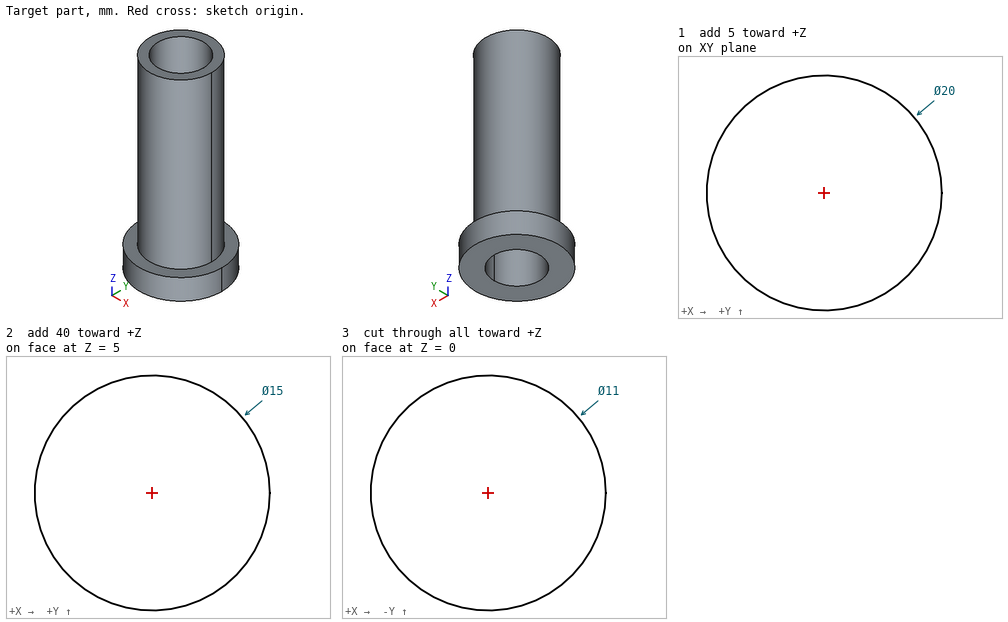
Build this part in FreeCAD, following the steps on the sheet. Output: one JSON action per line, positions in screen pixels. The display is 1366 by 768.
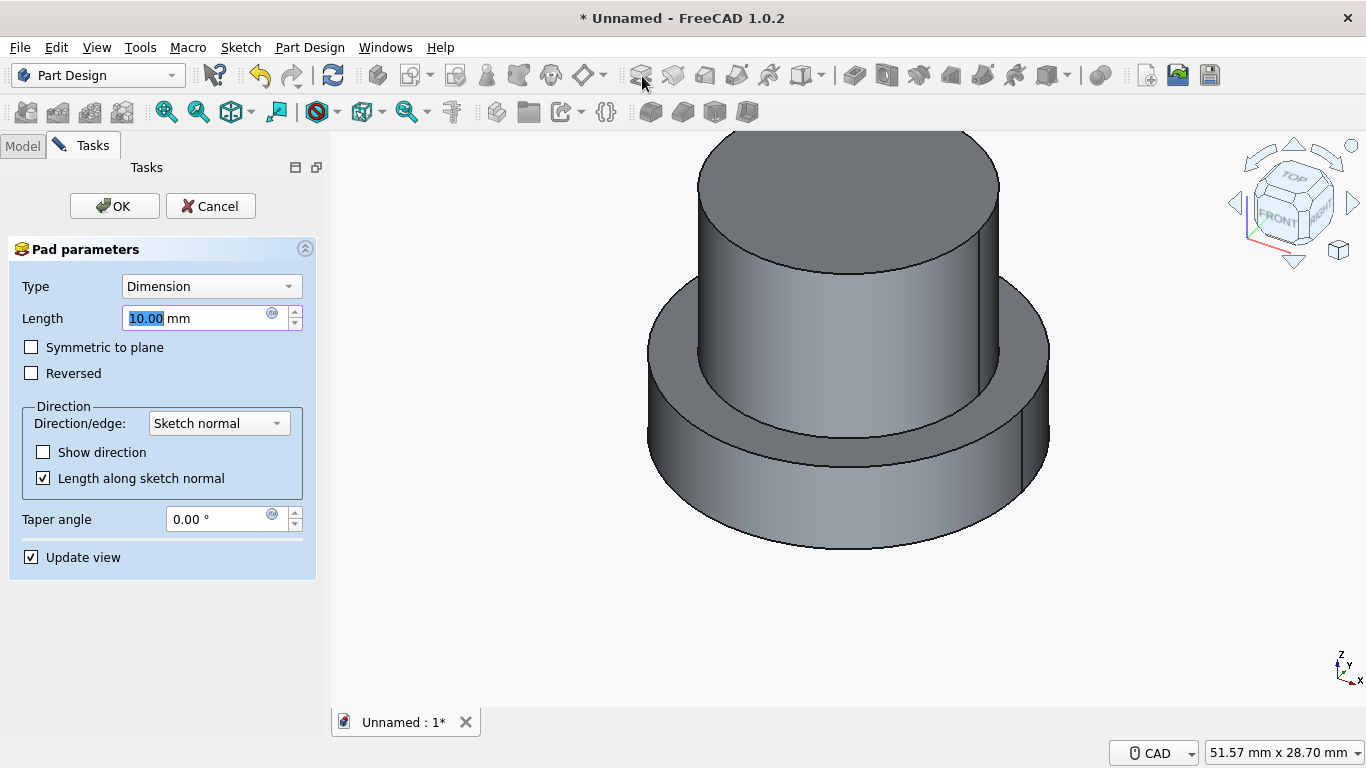
{"action": "type", "text": "40"}
{"action": "key", "text": "Tab"}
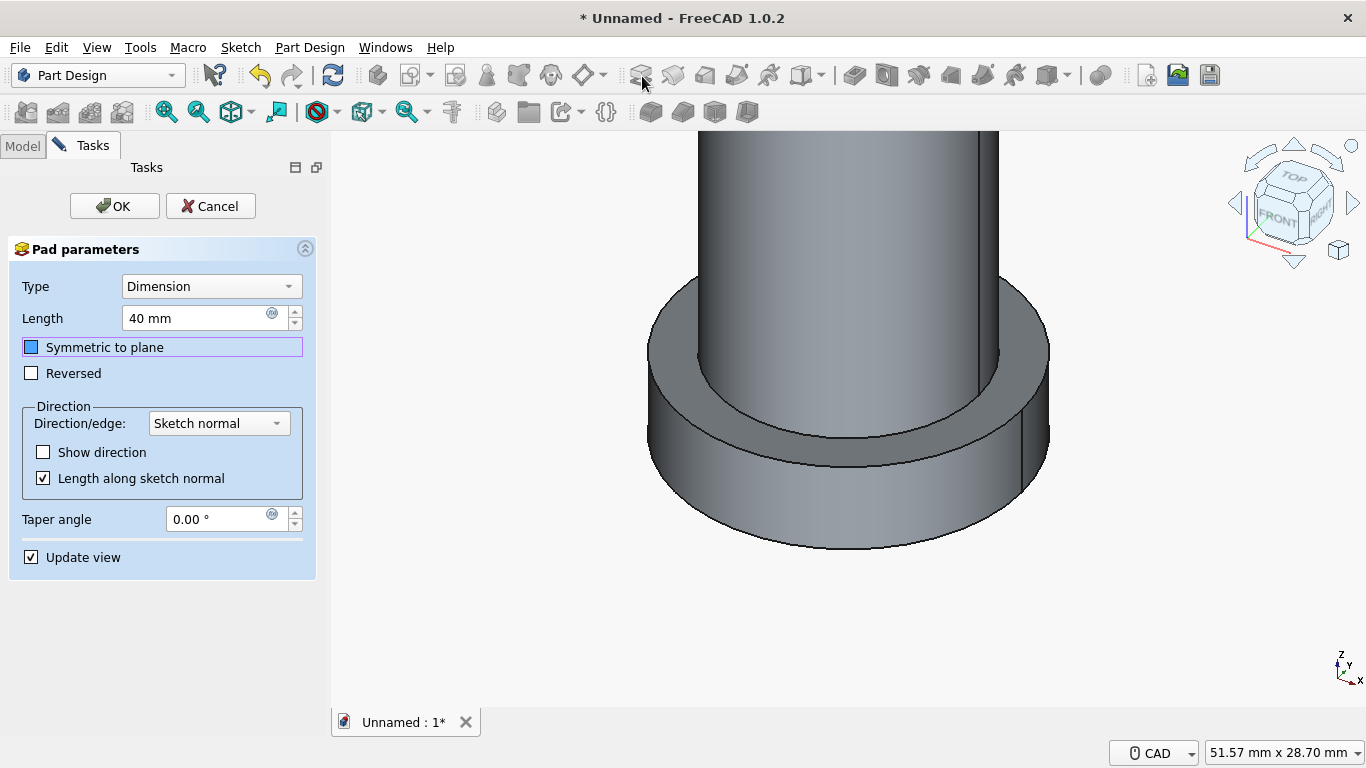
{"action": "left_click", "coordinate": [115, 206]}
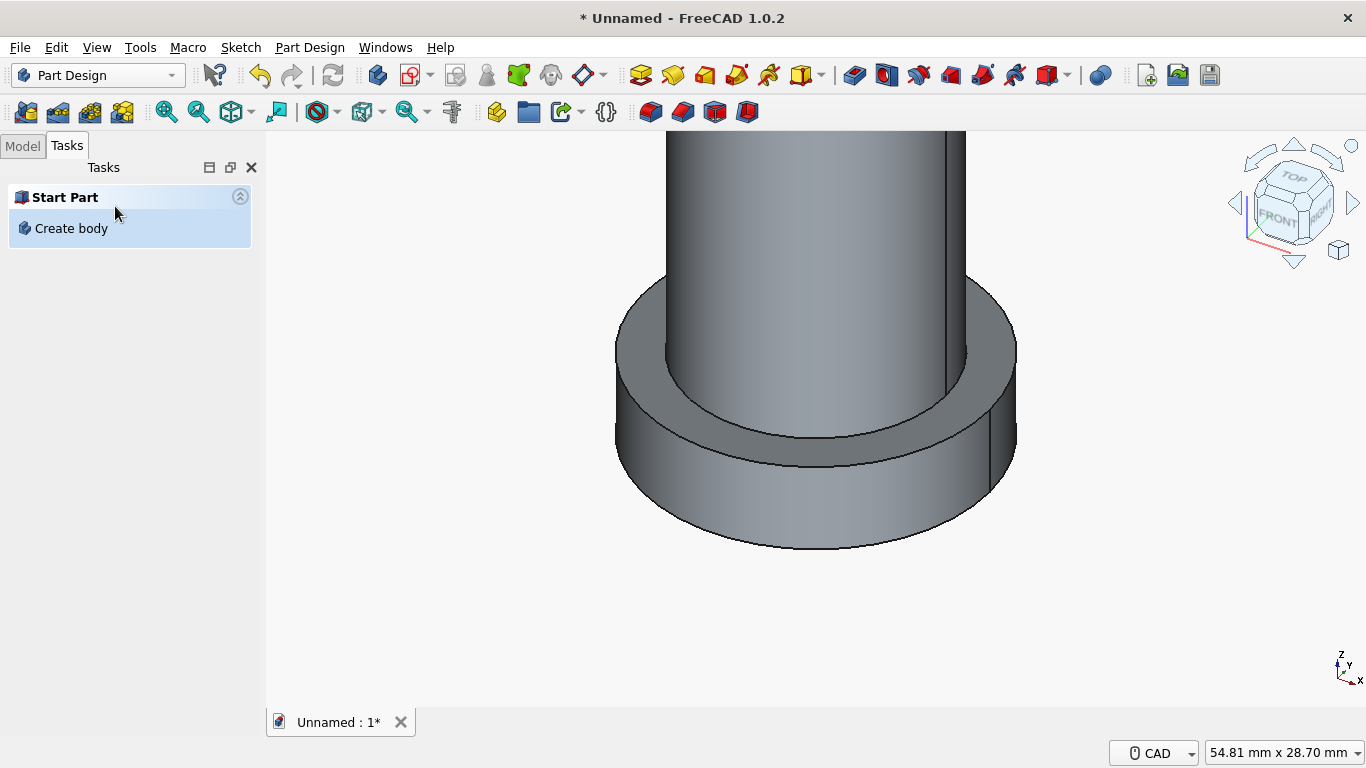
{"action": "left_click", "coordinate": [168, 112]}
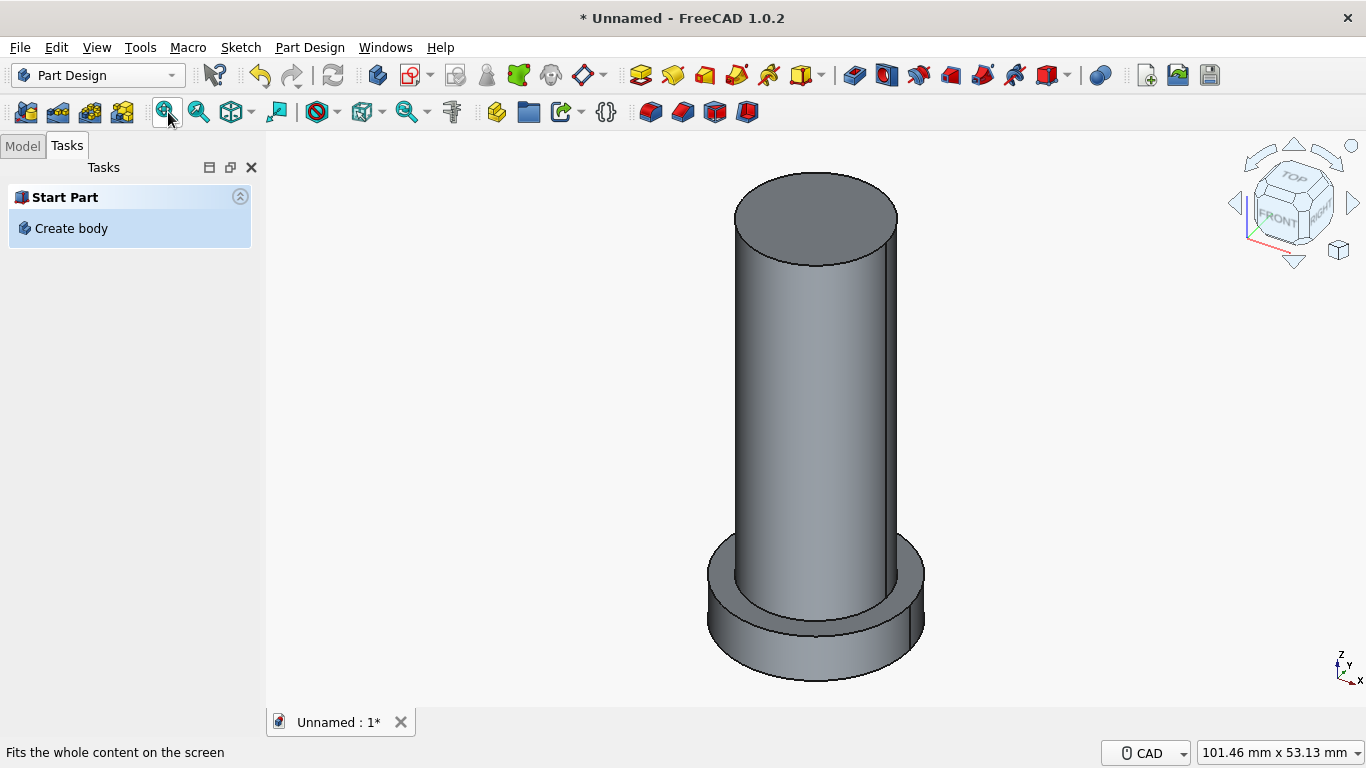
{"action": "key", "text": "5"}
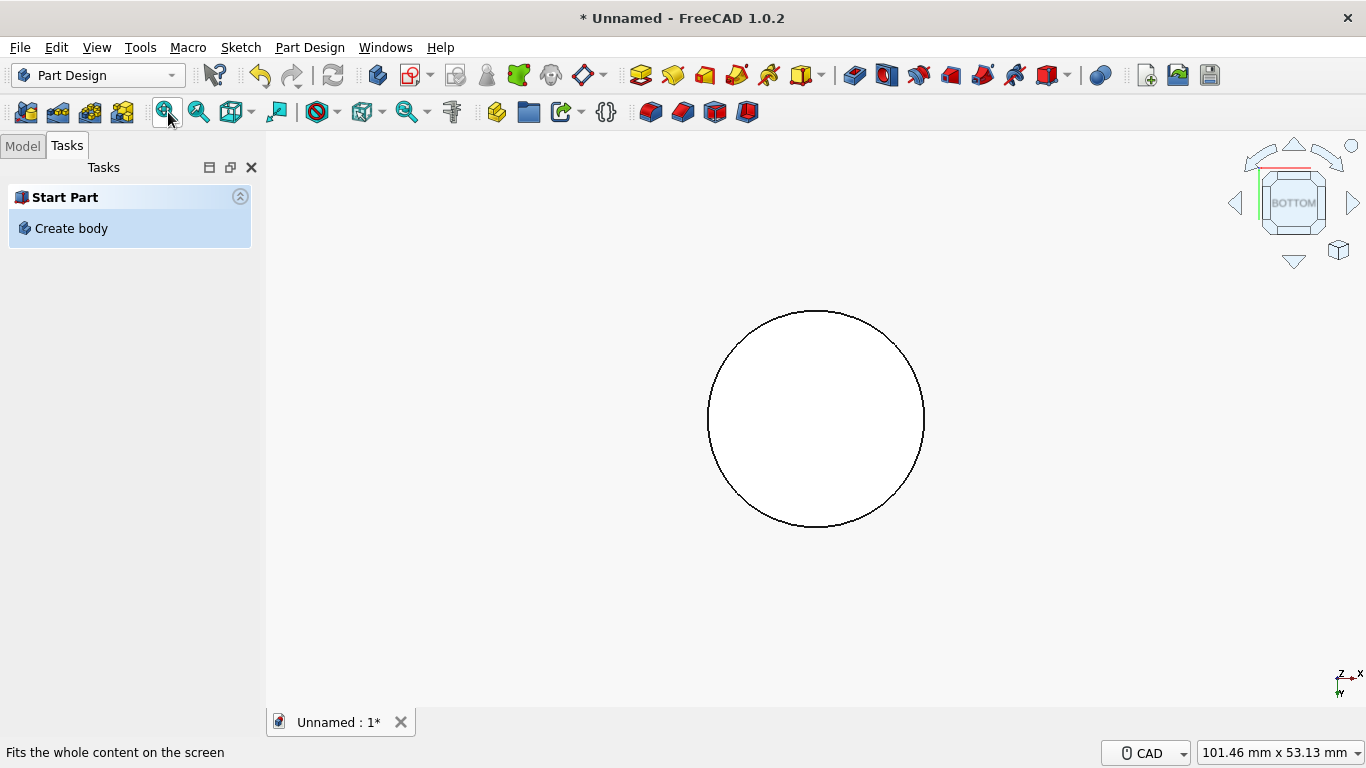
{"action": "key", "text": "v f"}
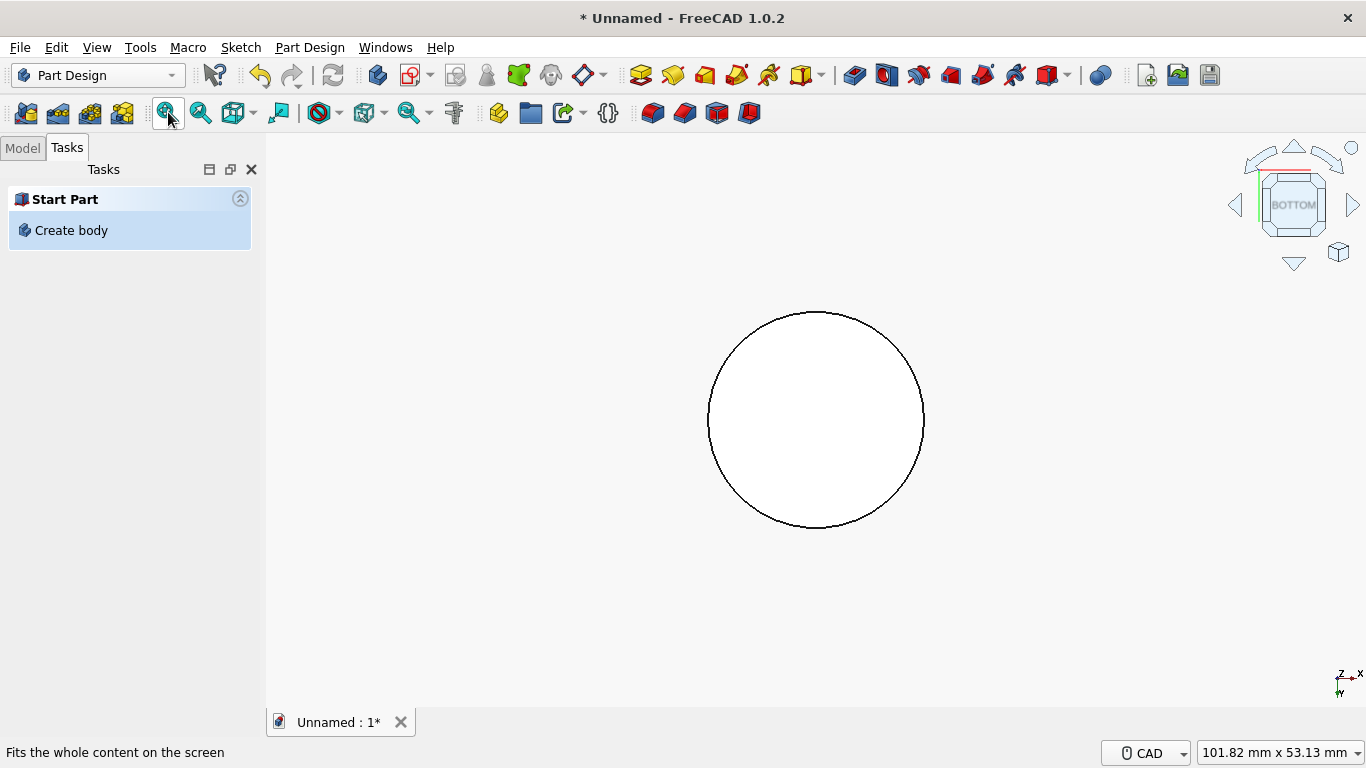
{"action": "left_click", "coordinate": [816, 419]}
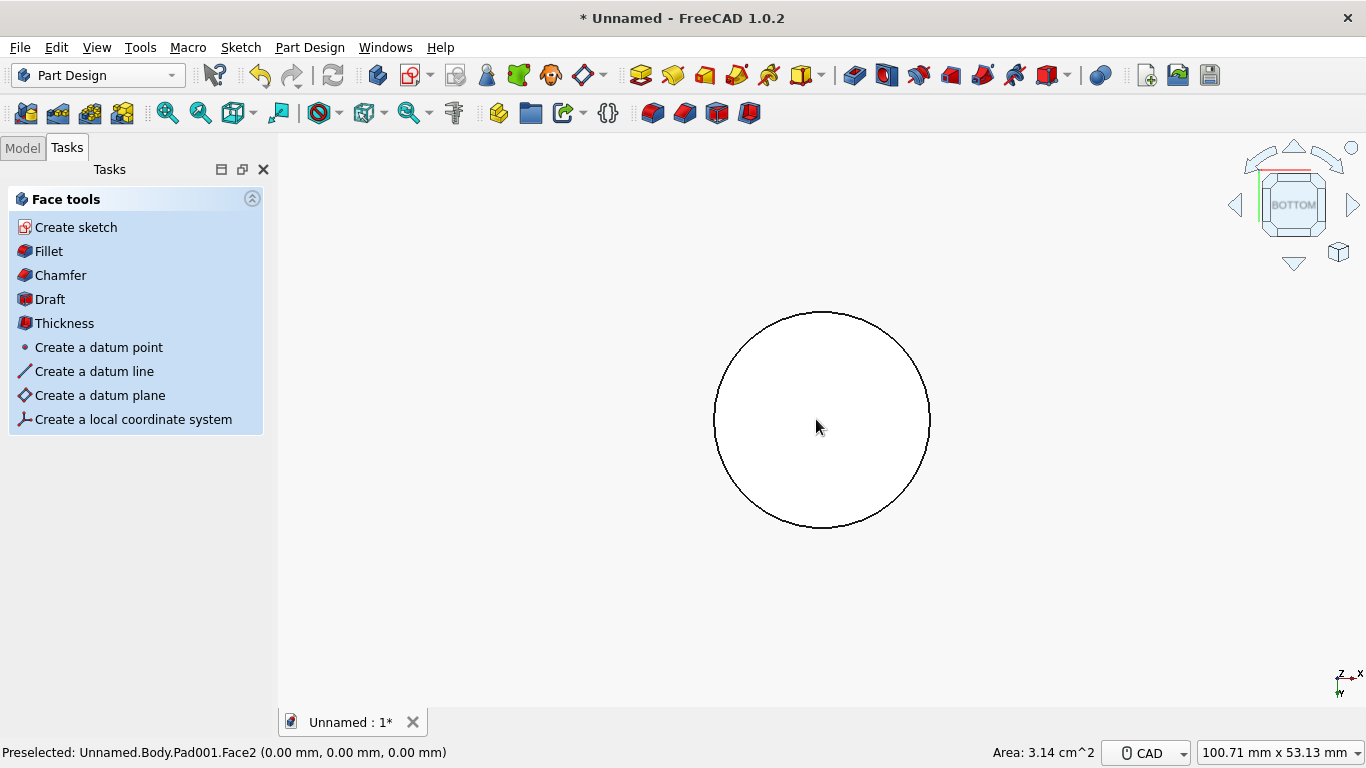
{"action": "left_click", "coordinate": [410, 76]}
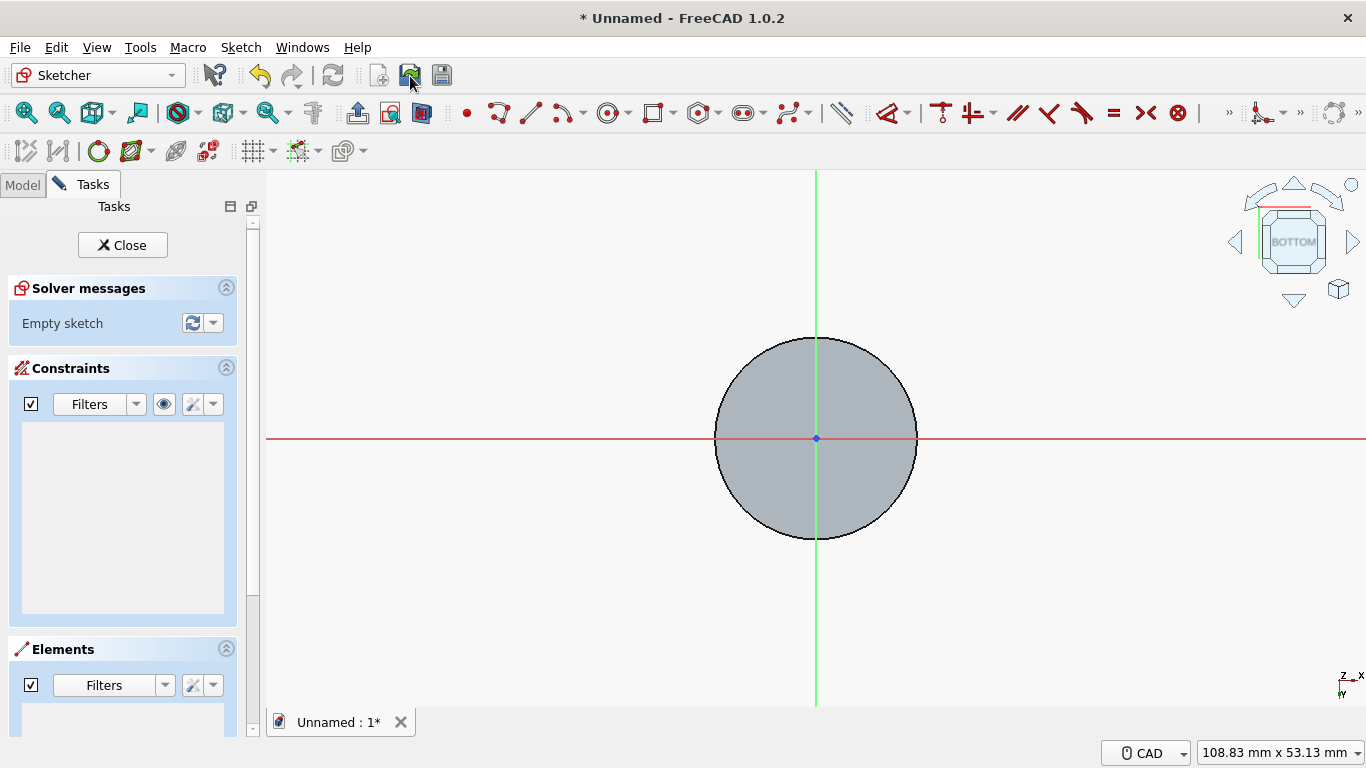
{"action": "scroll", "coordinate": [846, 438], "scroll_direction": "up", "scroll_amount": 6}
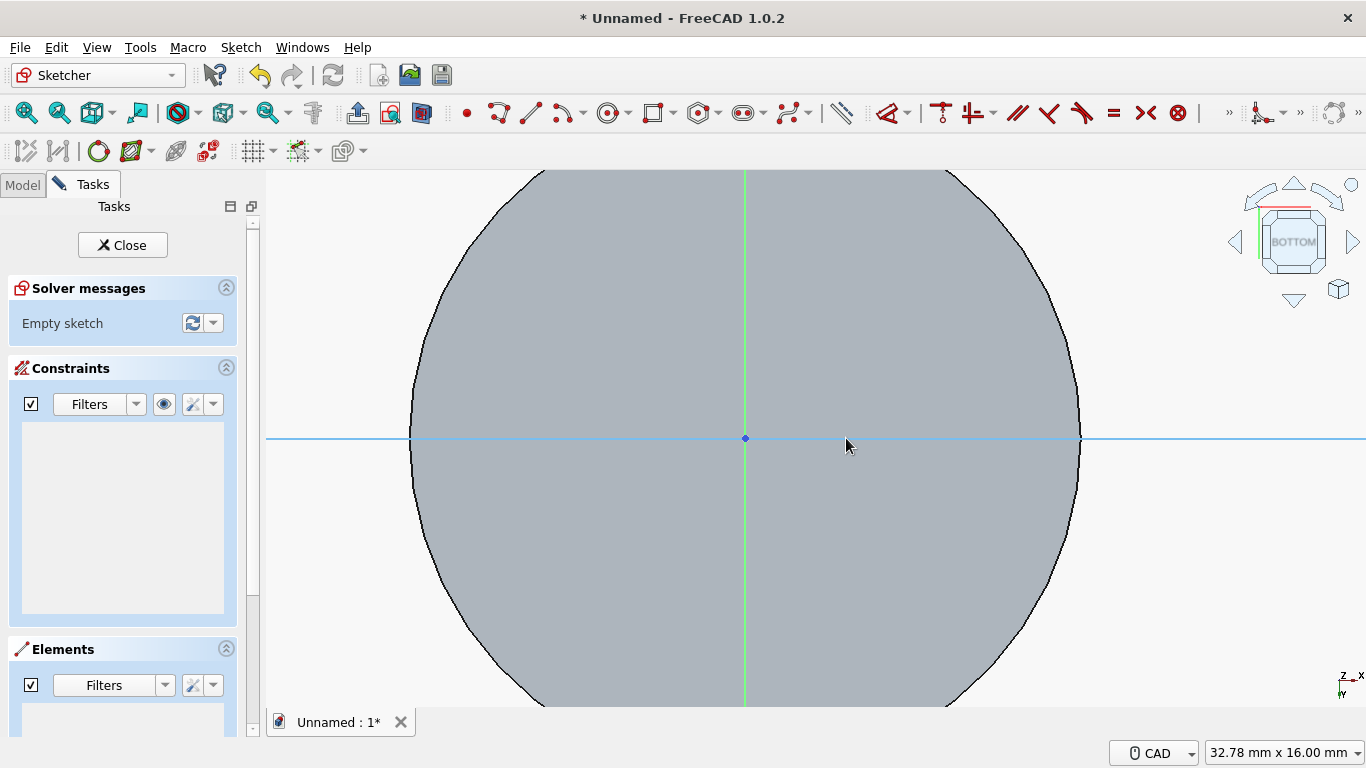
{"action": "left_click", "coordinate": [608, 114]}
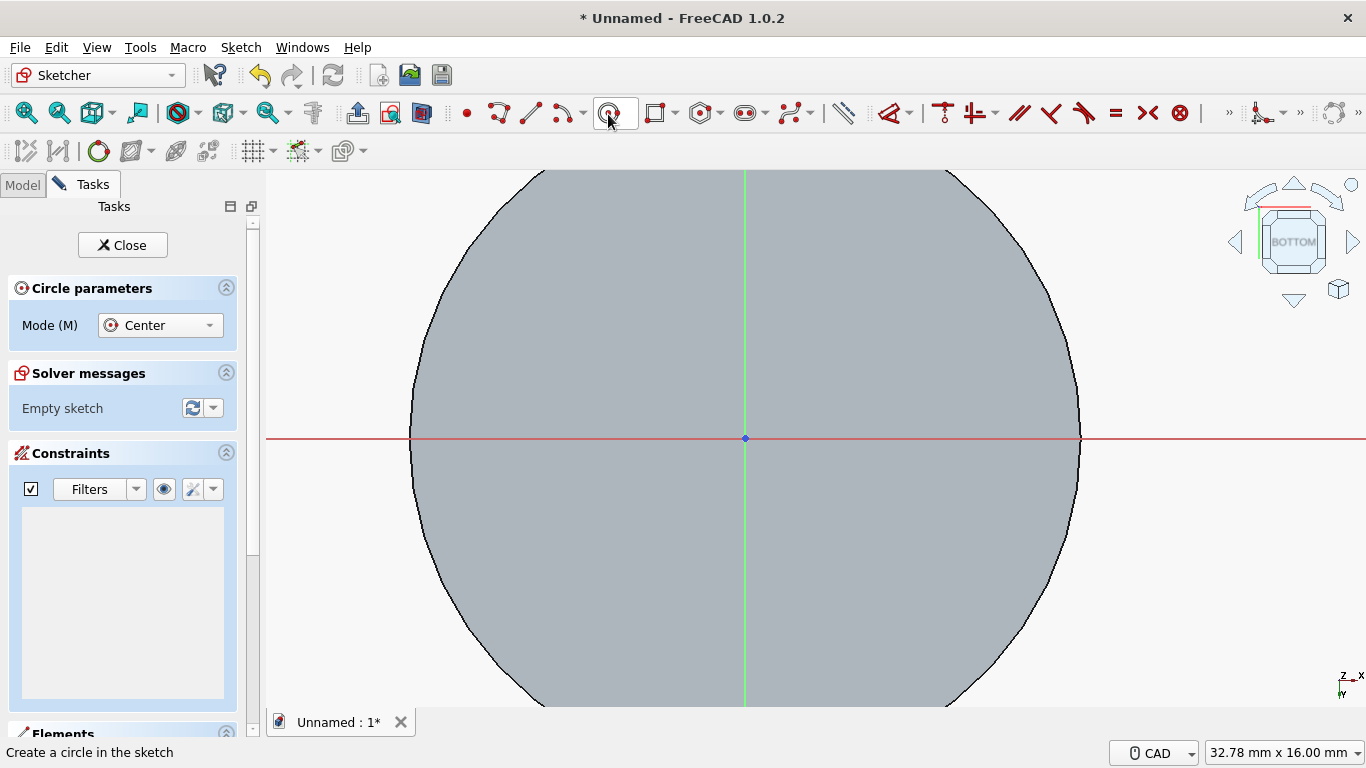
{"action": "left_click", "coordinate": [745, 438]}
{"action": "mouse_move", "coordinate": [876, 308]}